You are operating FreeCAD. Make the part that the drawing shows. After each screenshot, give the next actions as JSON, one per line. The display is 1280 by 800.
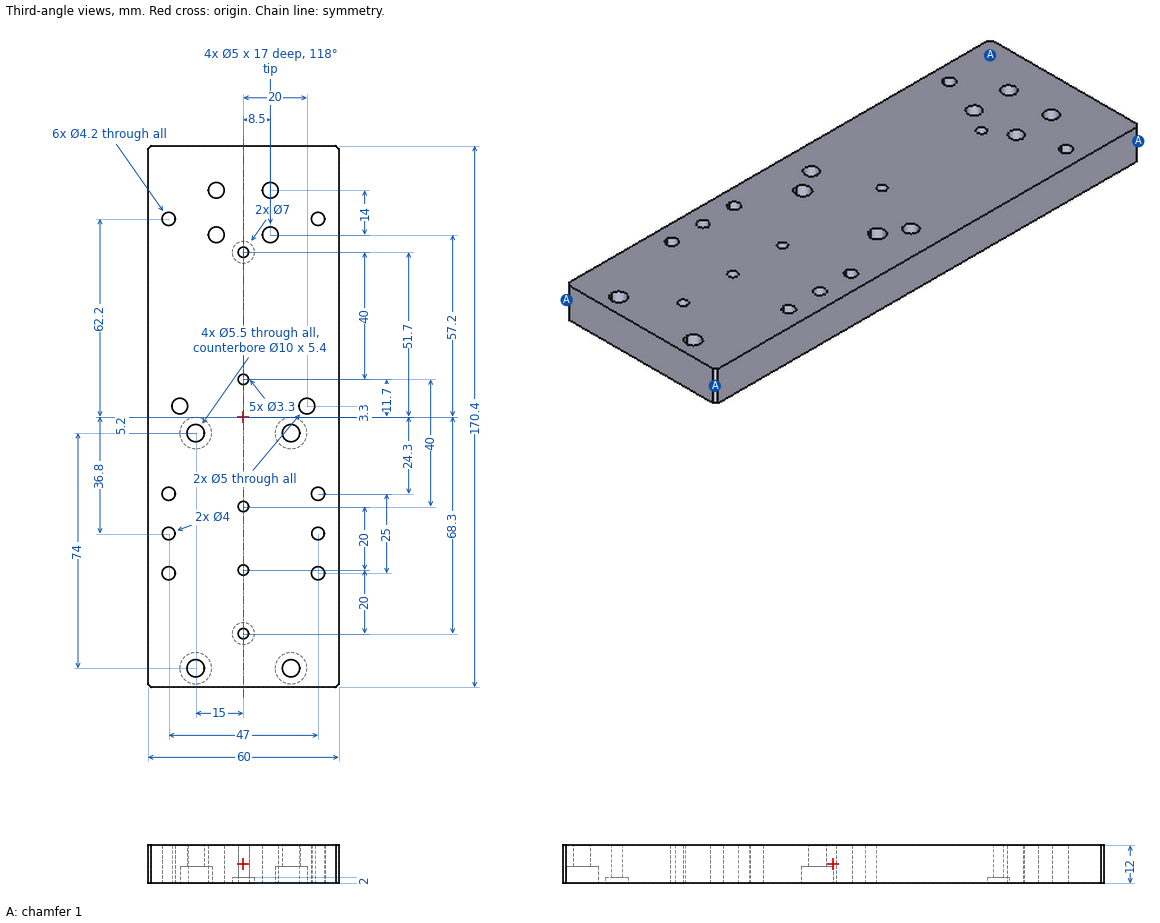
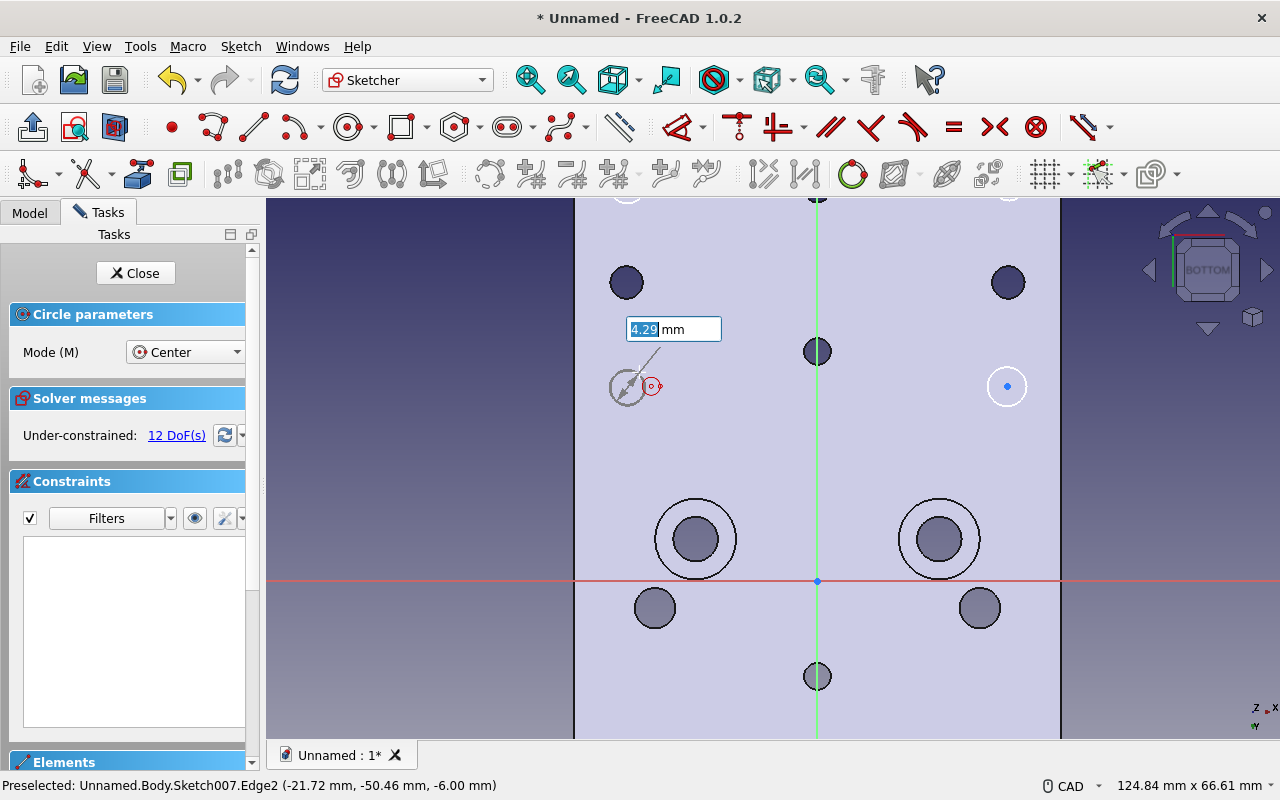
{"action": "left_click", "coordinate": [639, 372]}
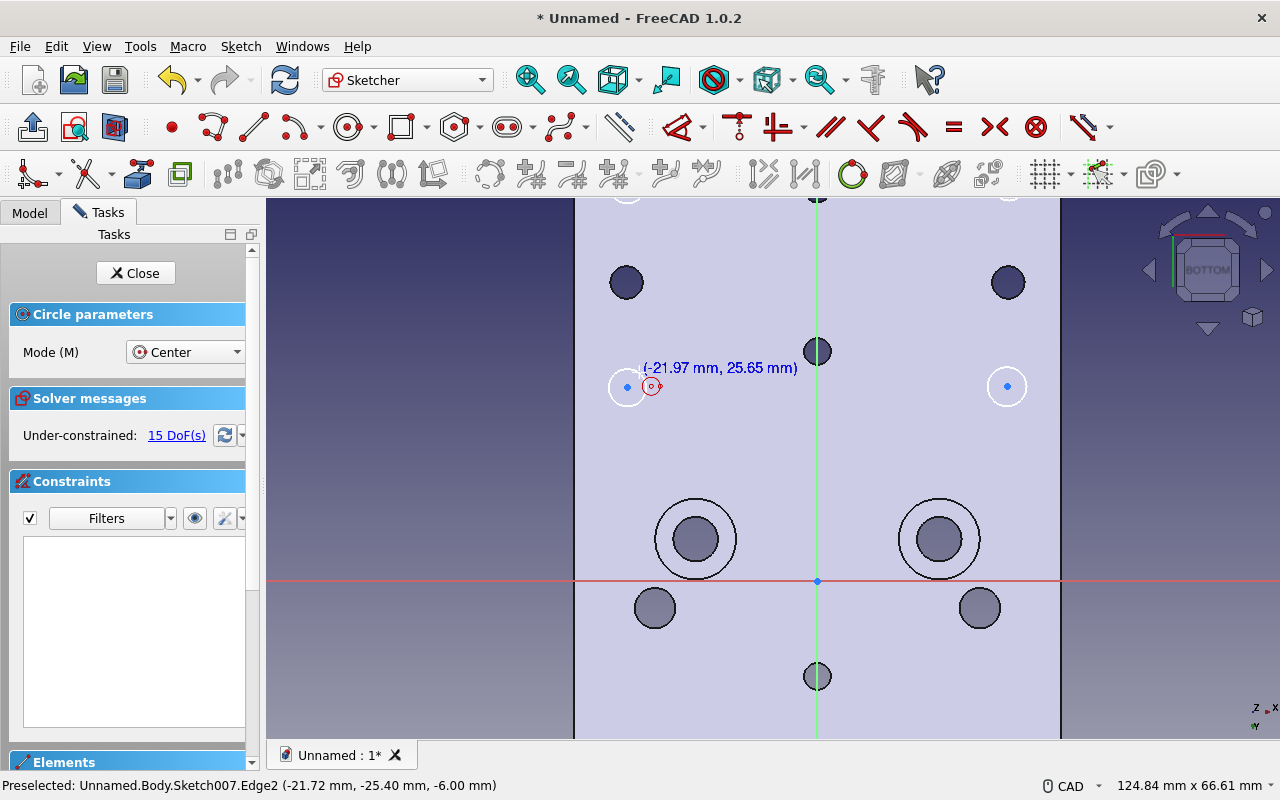
{"action": "scroll", "coordinate": [639, 372], "scroll_direction": "down", "scroll_amount": 5}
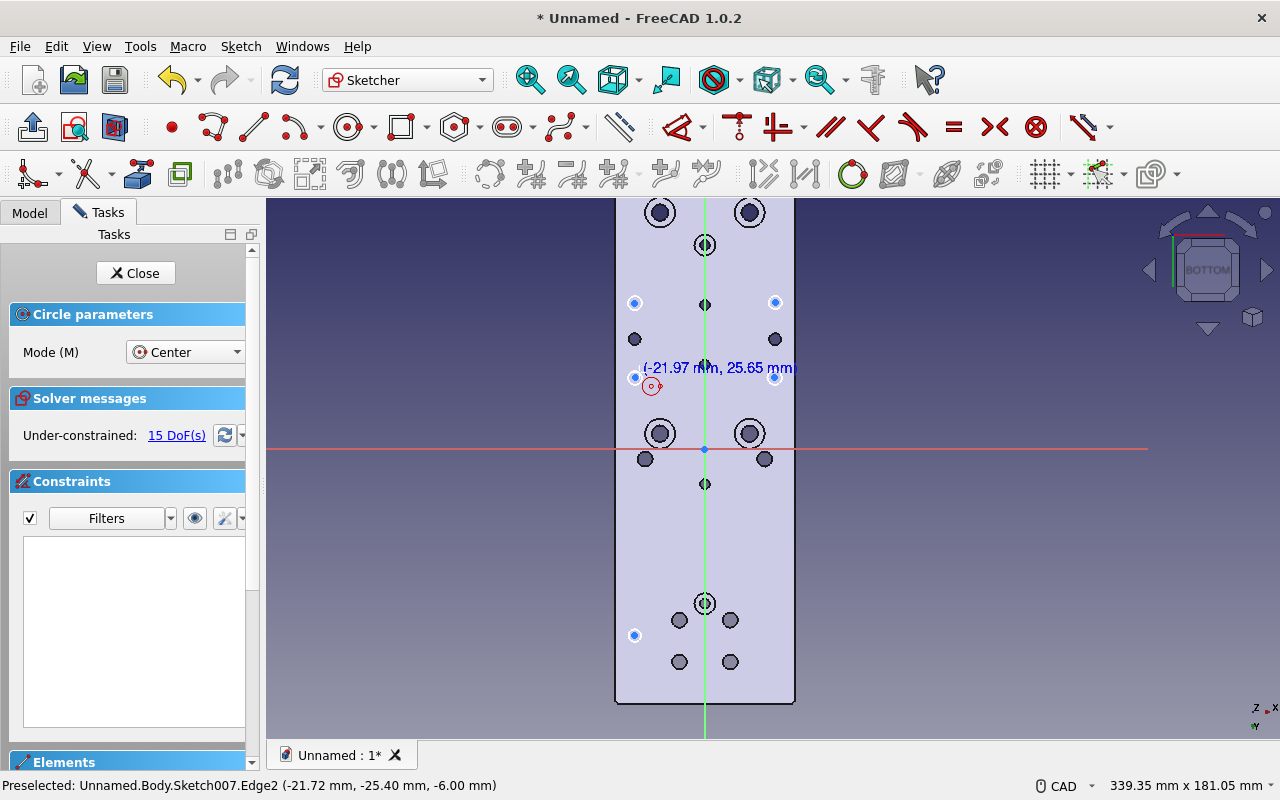
{"action": "scroll", "coordinate": [775, 635], "scroll_direction": "up", "scroll_amount": 7}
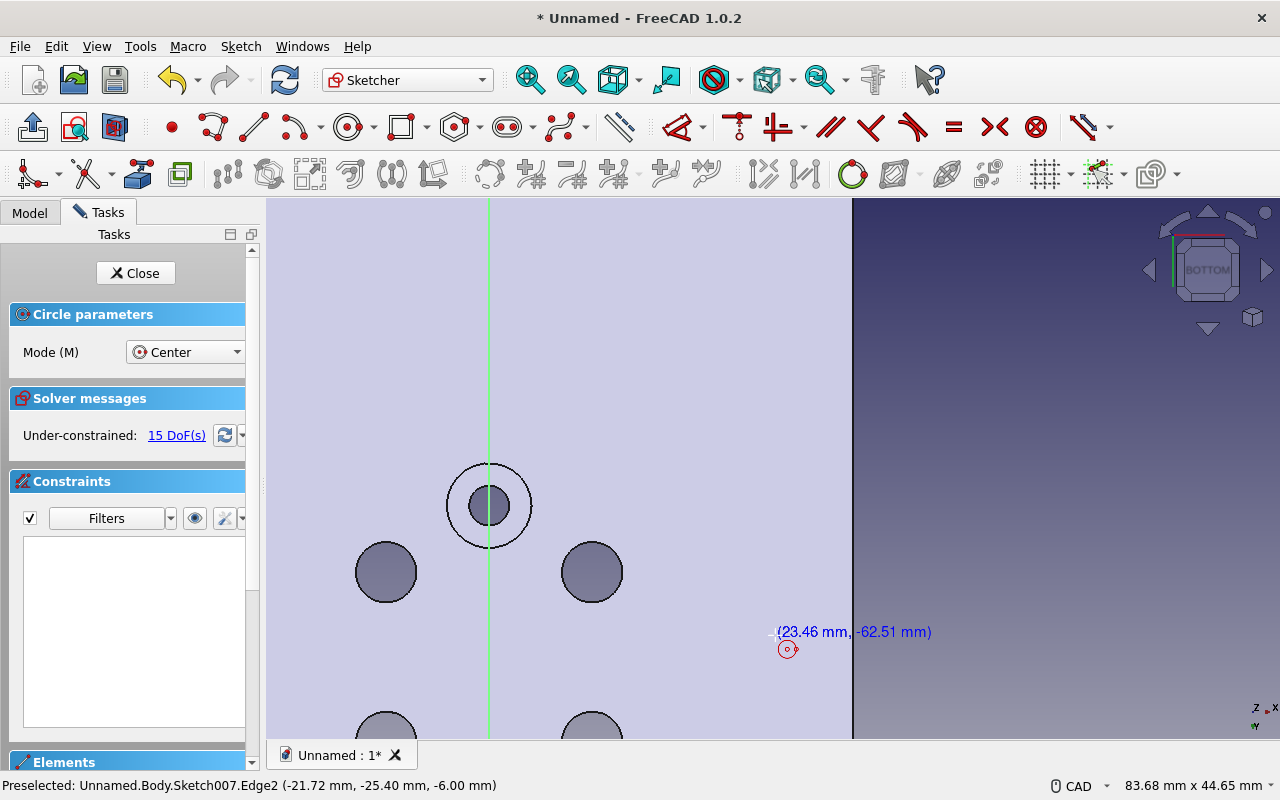
{"action": "scroll", "coordinate": [775, 636], "scroll_direction": "down", "scroll_amount": 7}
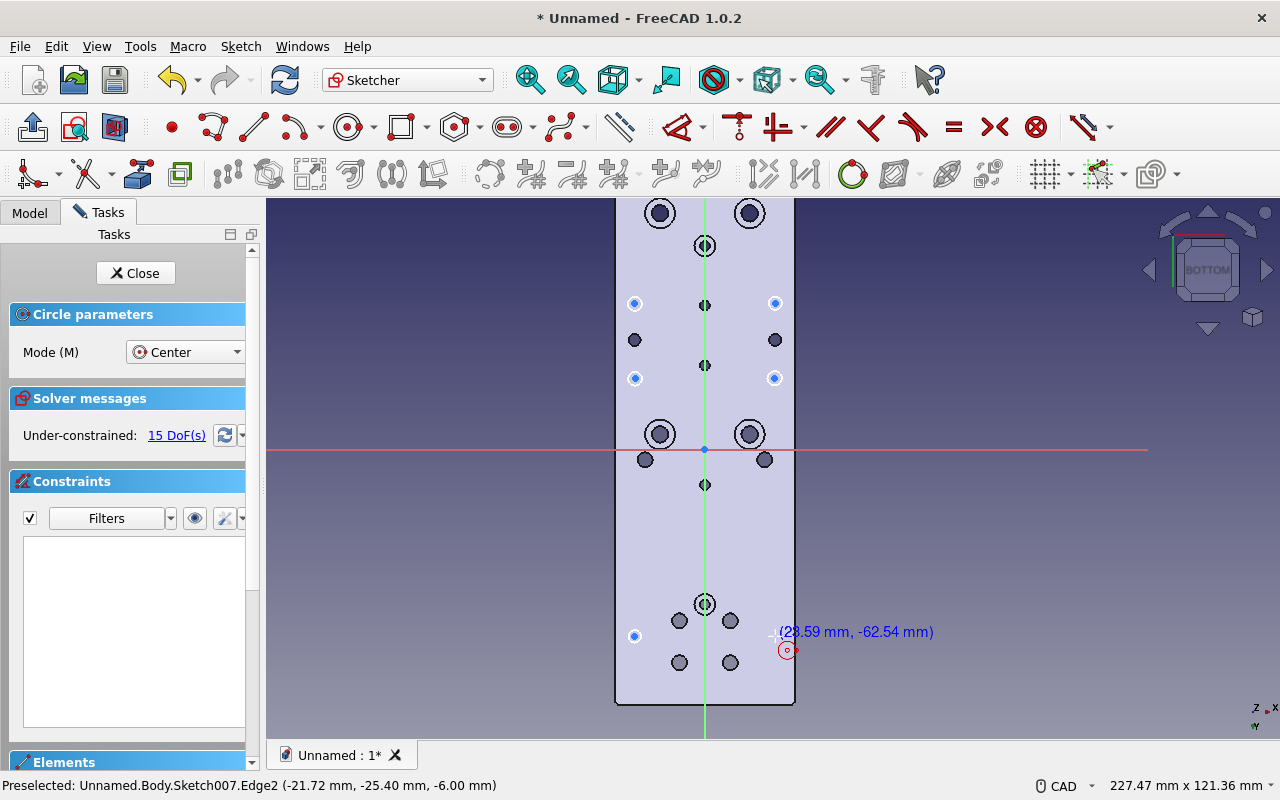
{"action": "left_click", "coordinate": [775, 636]}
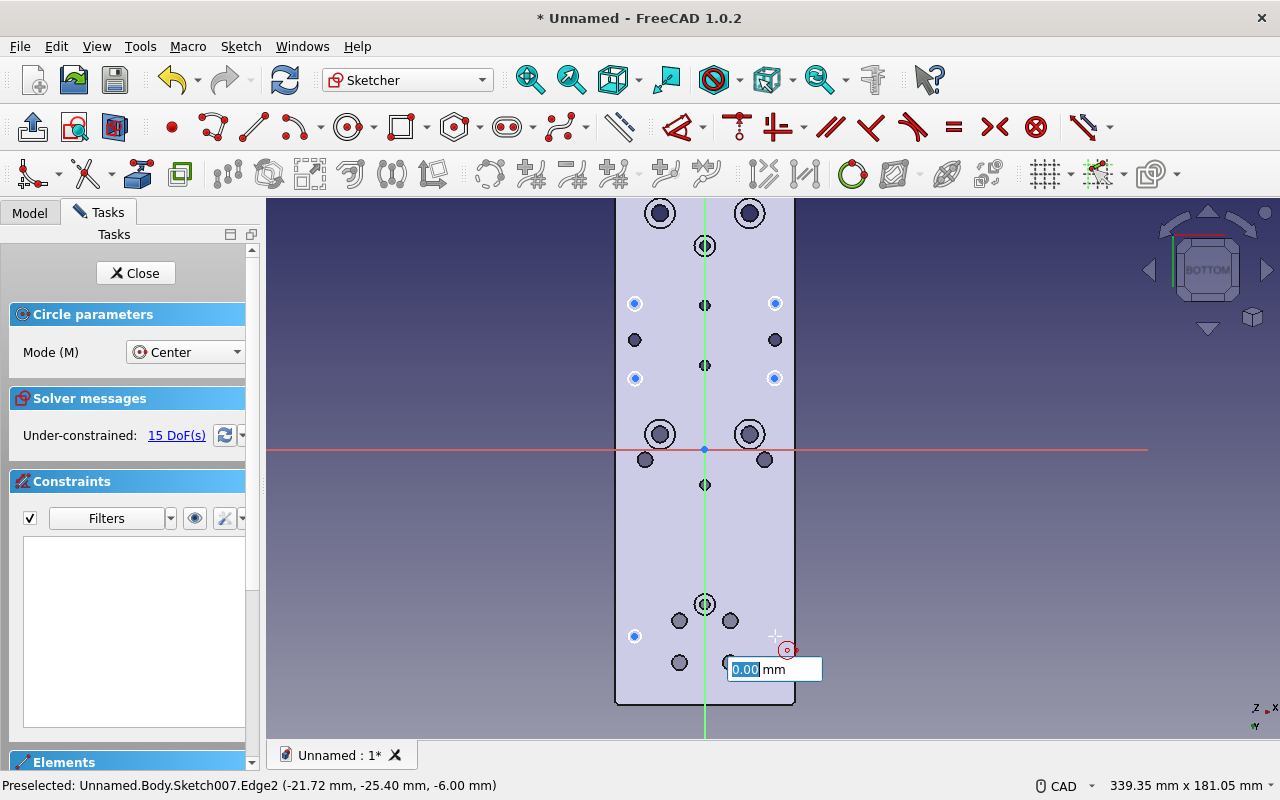
{"action": "scroll", "coordinate": [780, 631], "scroll_direction": "up", "scroll_amount": 5}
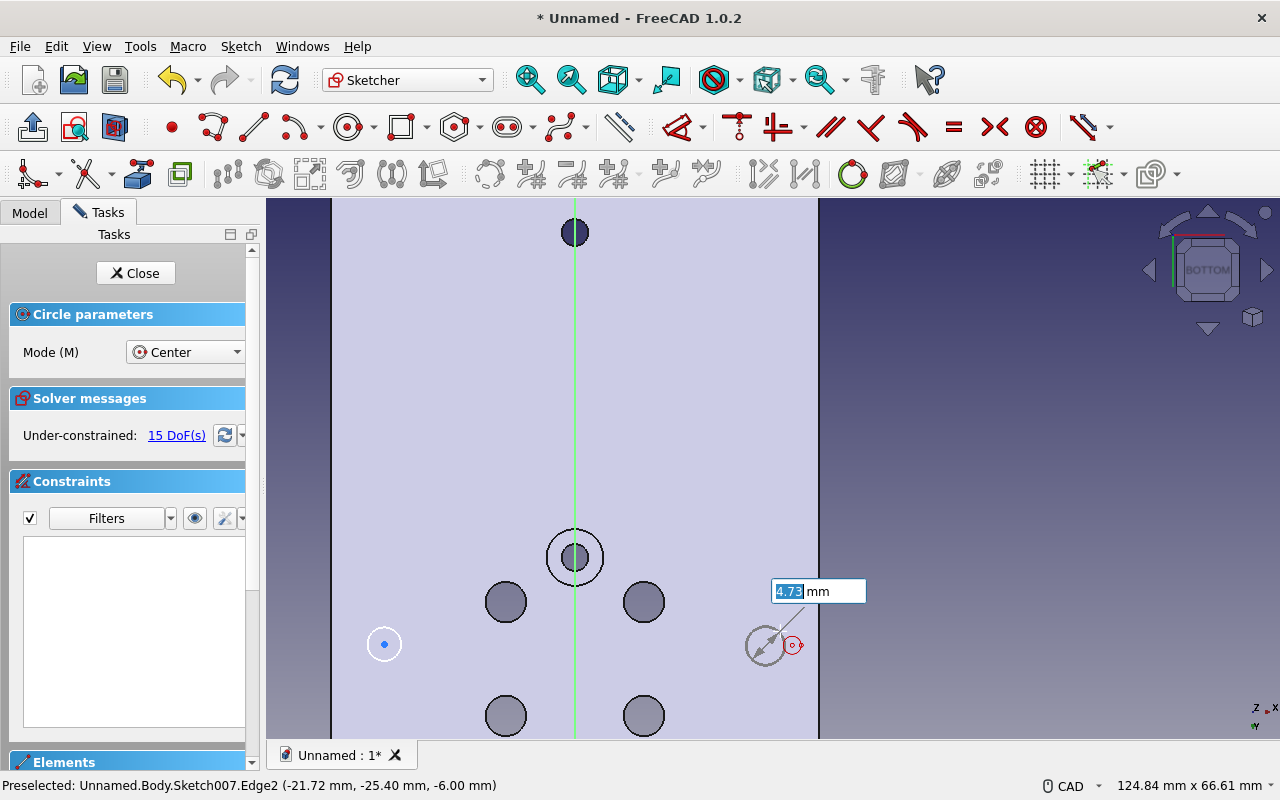
{"action": "left_click", "coordinate": [778, 631]}
{"action": "key", "text": "Escape"}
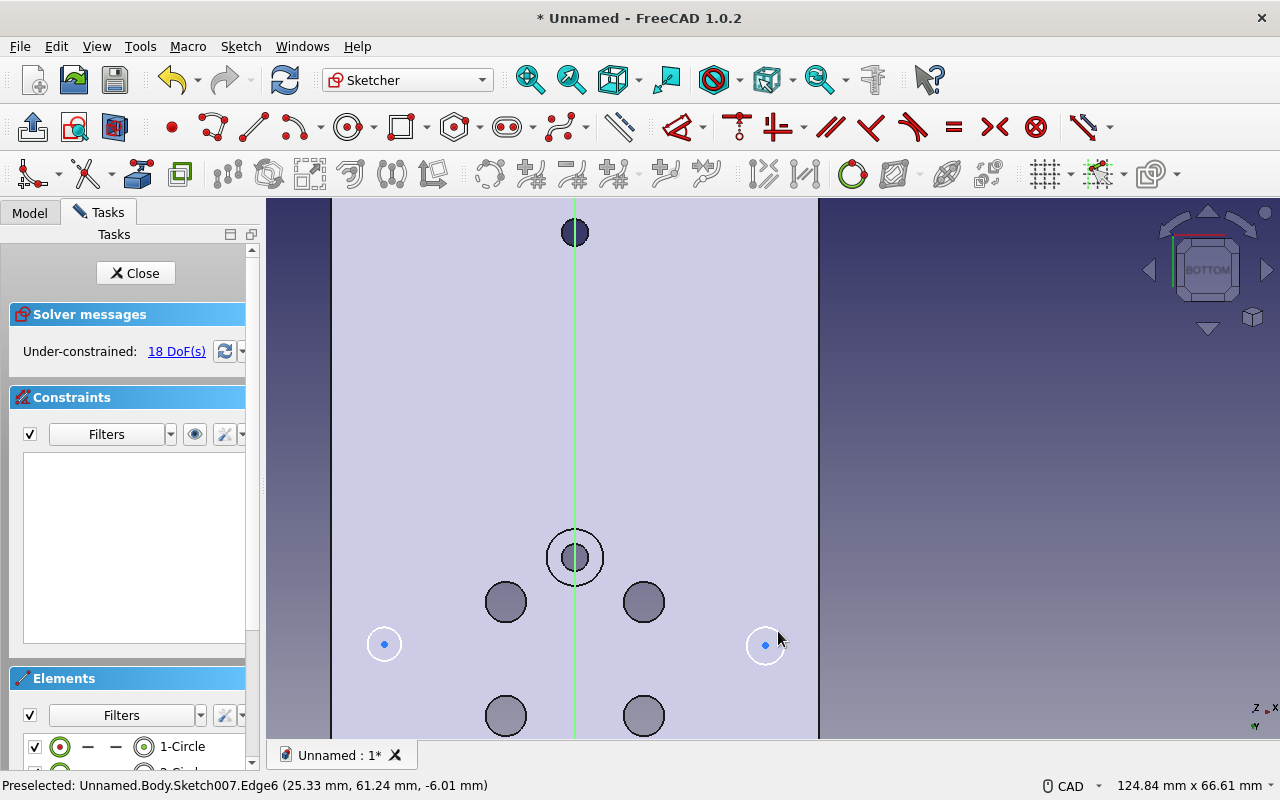
{"action": "left_click", "coordinate": [396, 632]}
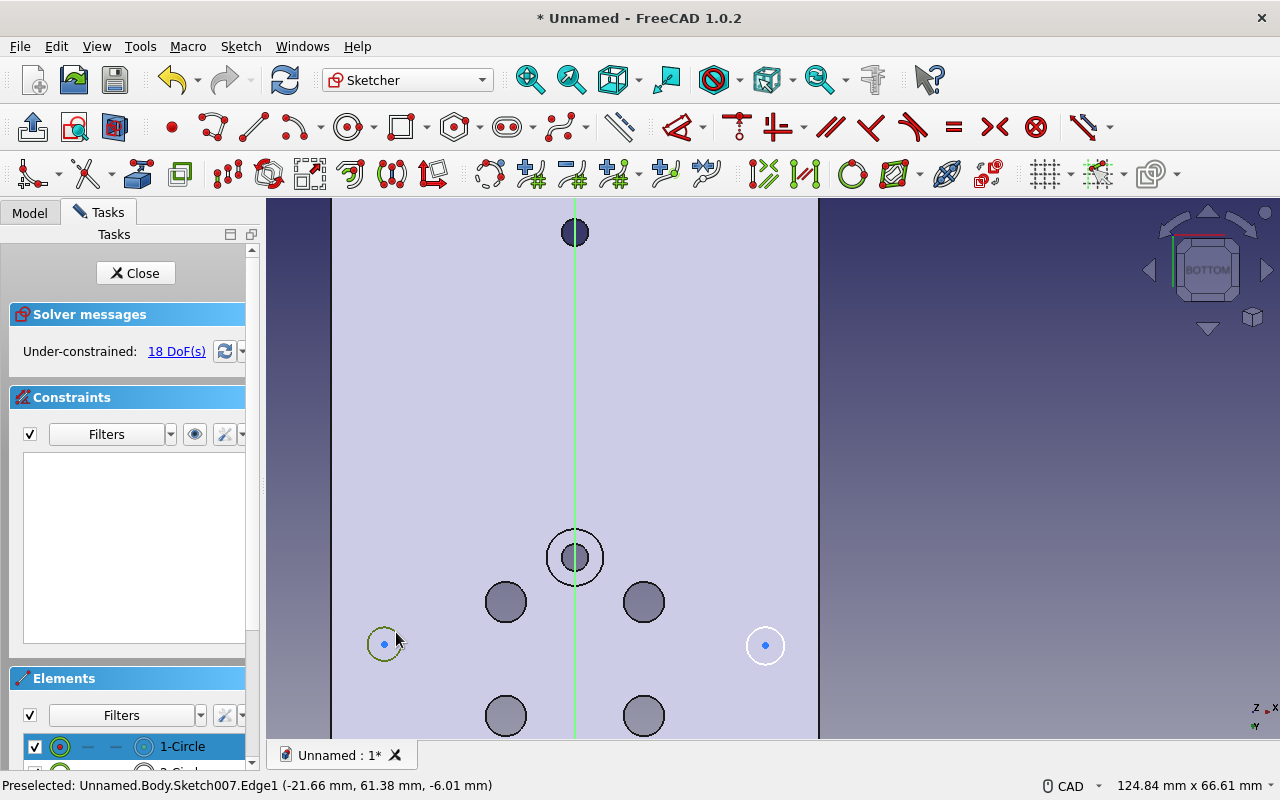
{"action": "scroll", "coordinate": [780, 631], "scroll_direction": "down", "scroll_amount": 5}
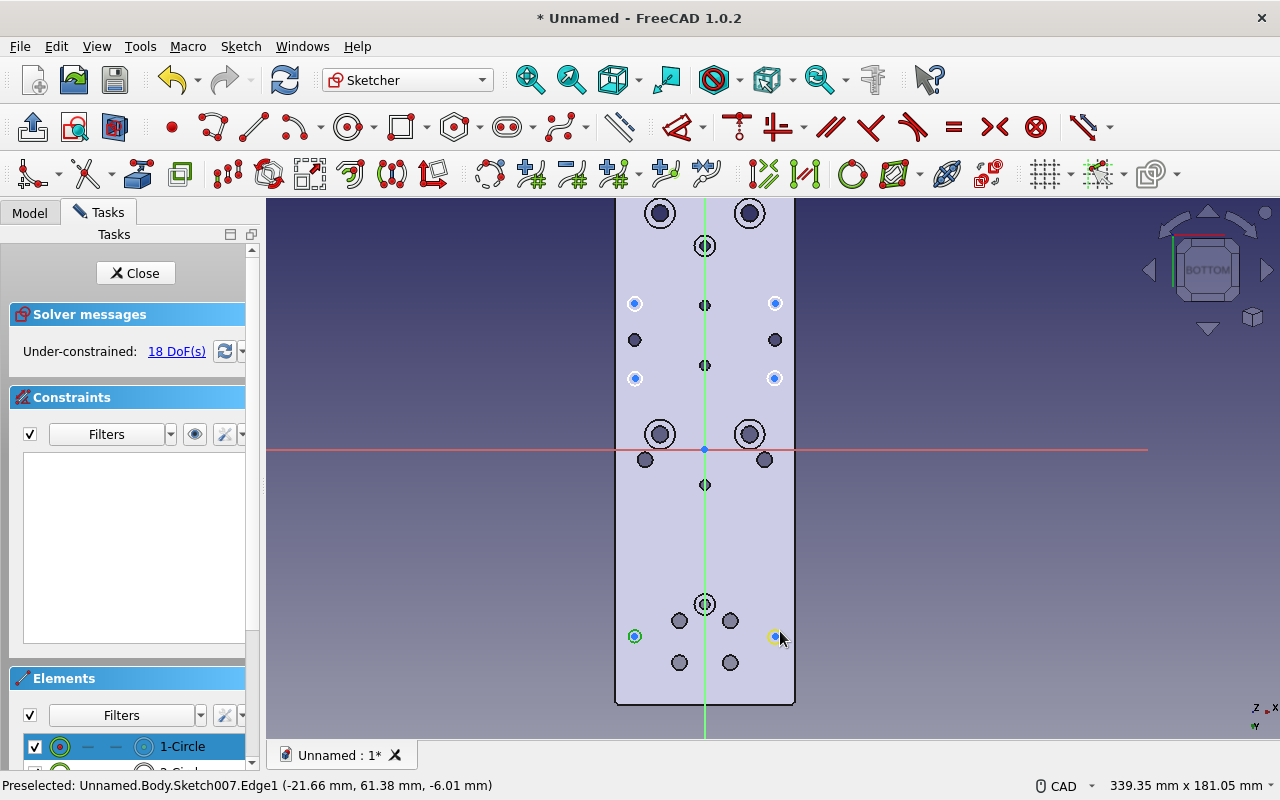
{"action": "scroll", "coordinate": [780, 373], "scroll_direction": "up", "scroll_amount": 4}